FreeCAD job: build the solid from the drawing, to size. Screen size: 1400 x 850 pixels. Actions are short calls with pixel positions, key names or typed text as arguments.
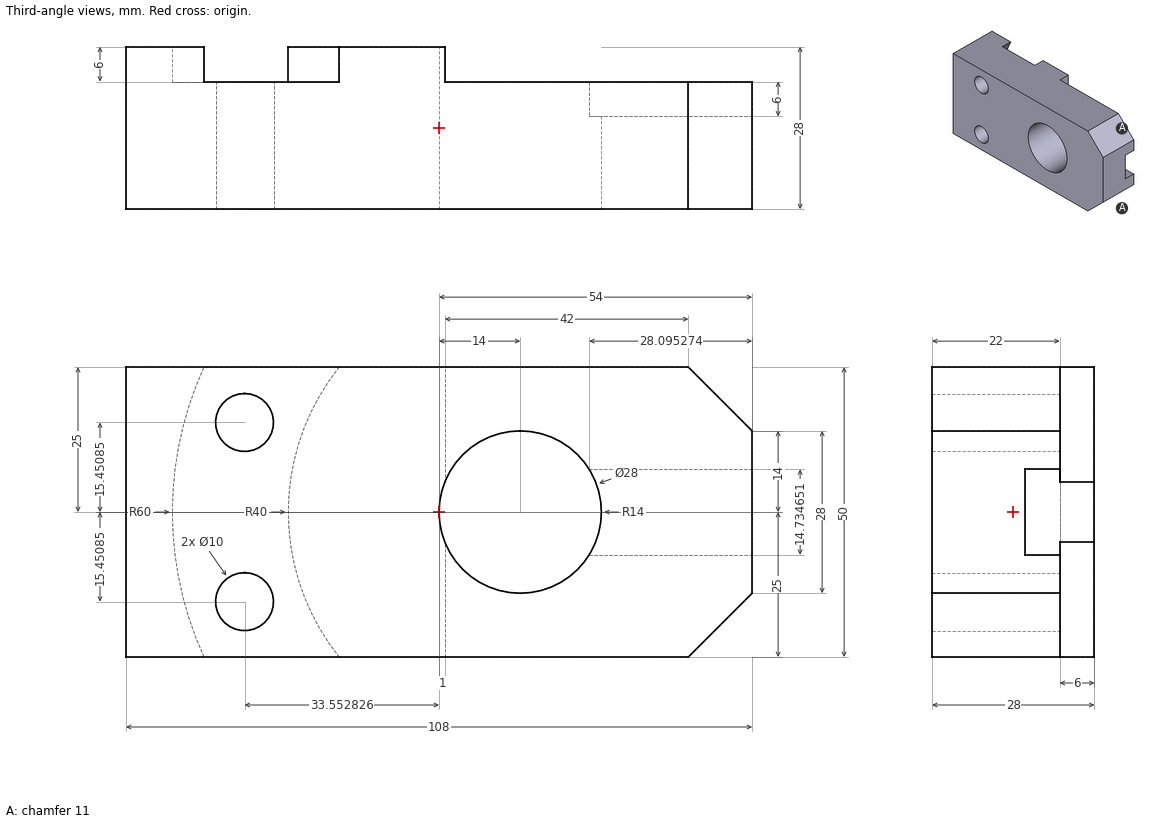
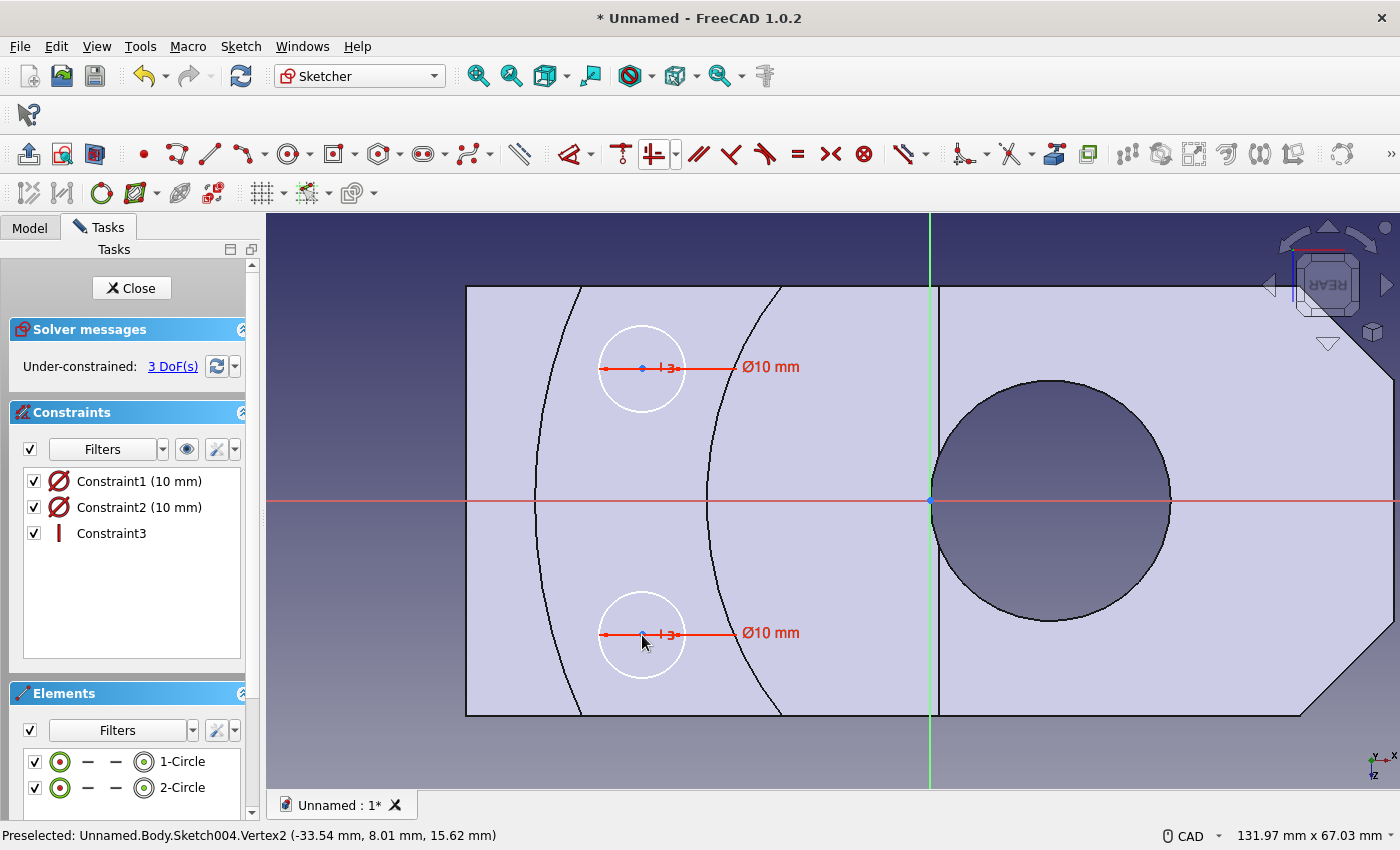
click(568, 154)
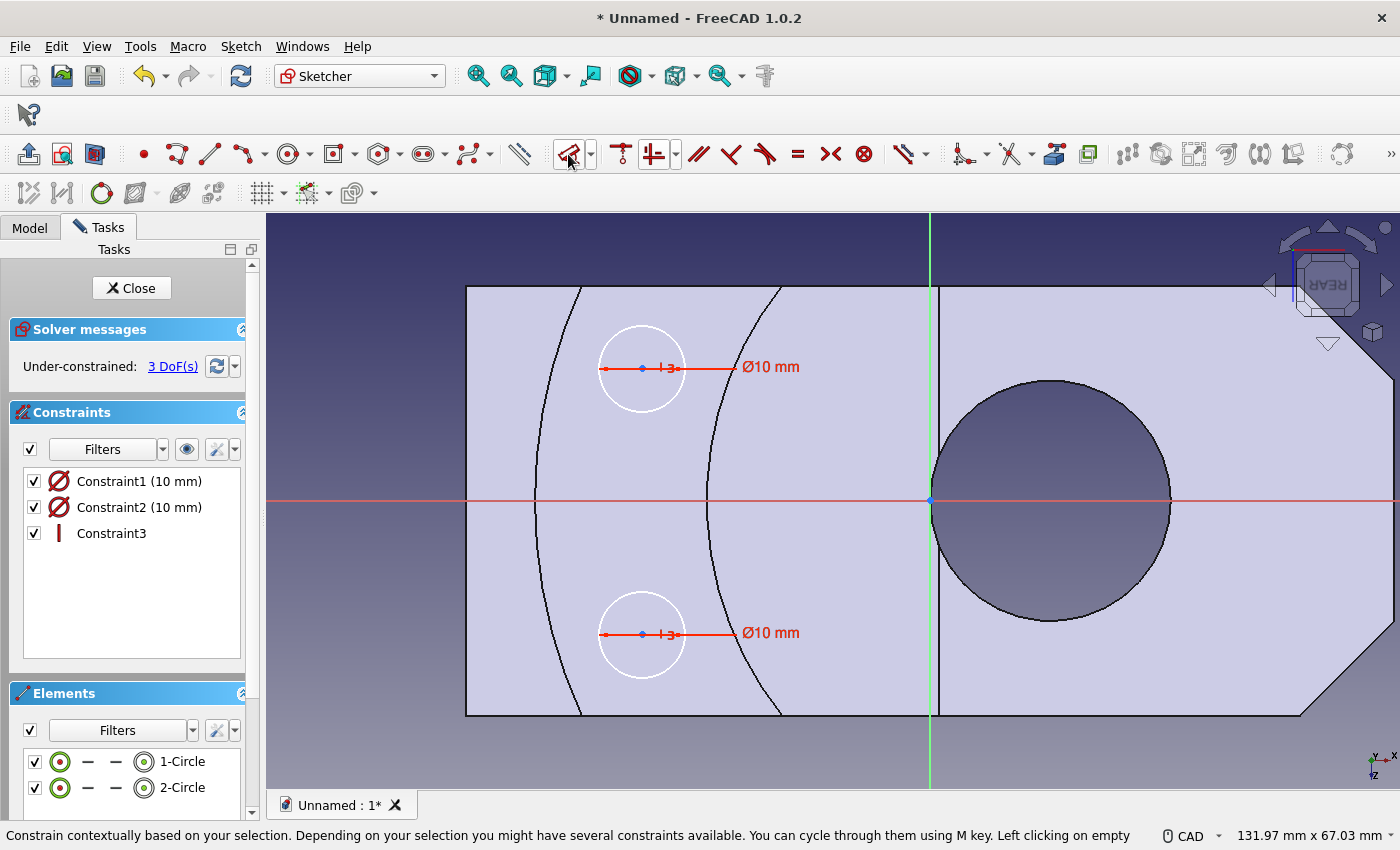
click(642, 369)
click(964, 435)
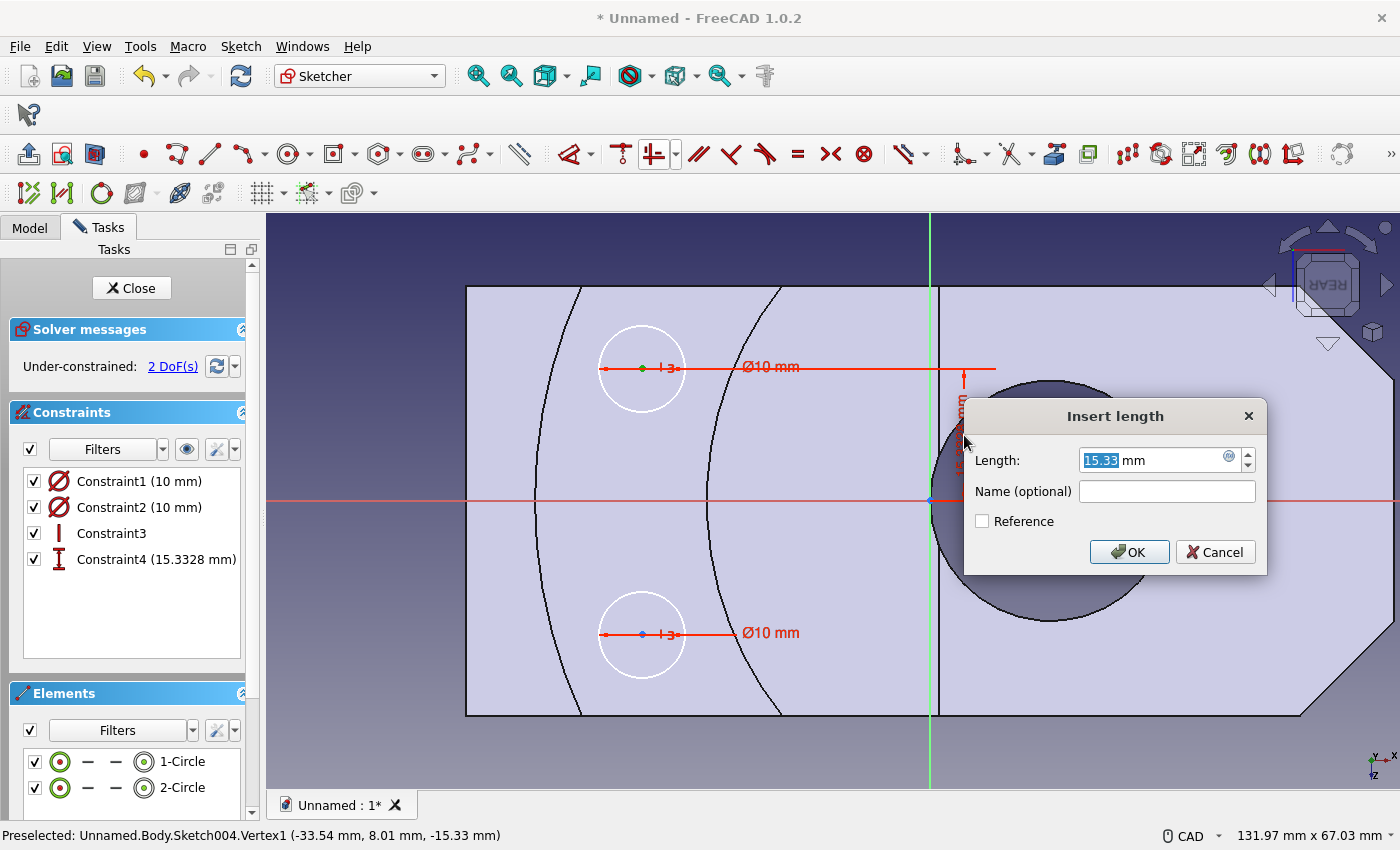
text(15.45085)
key(Return)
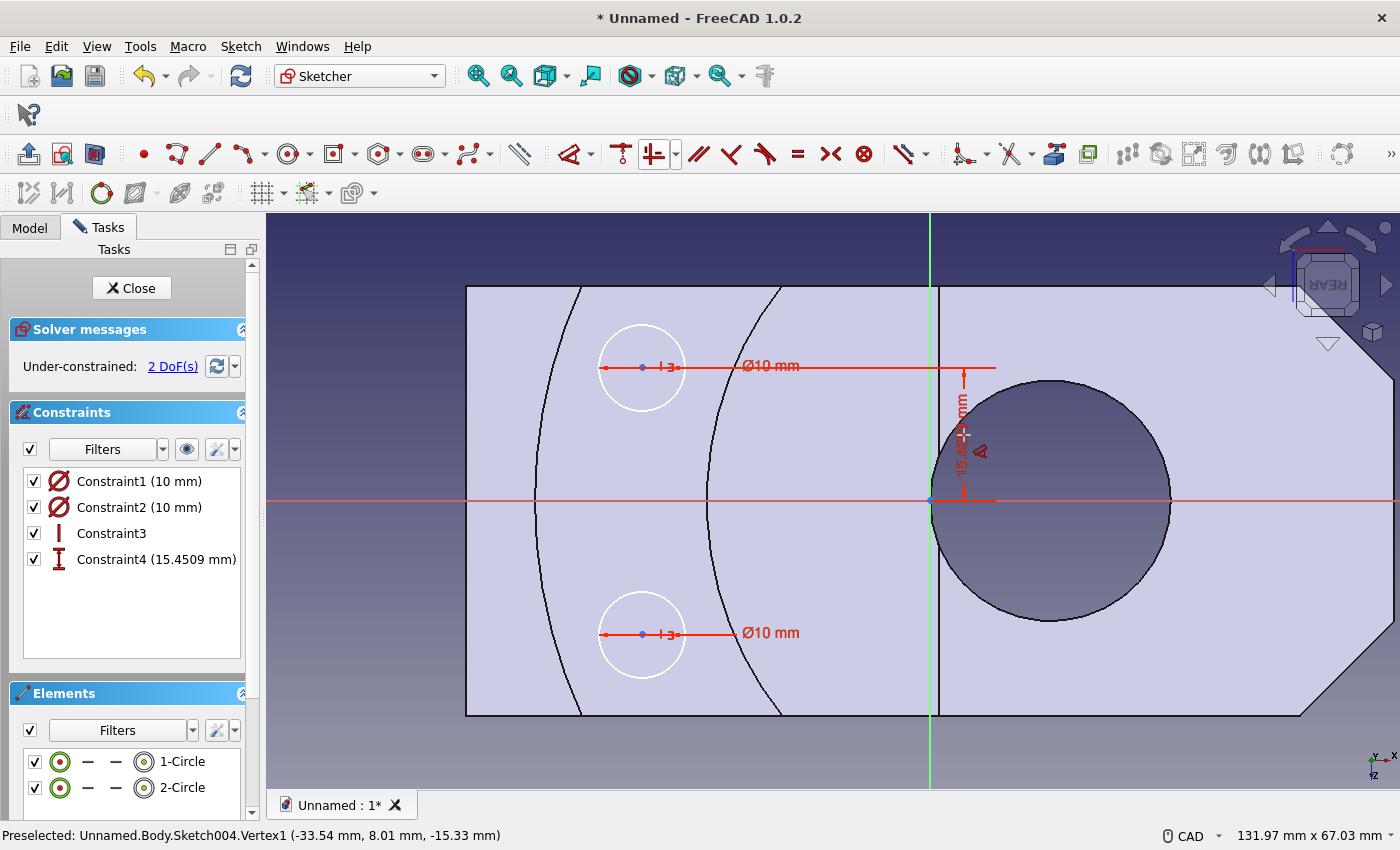
click(642, 635)
click(964, 568)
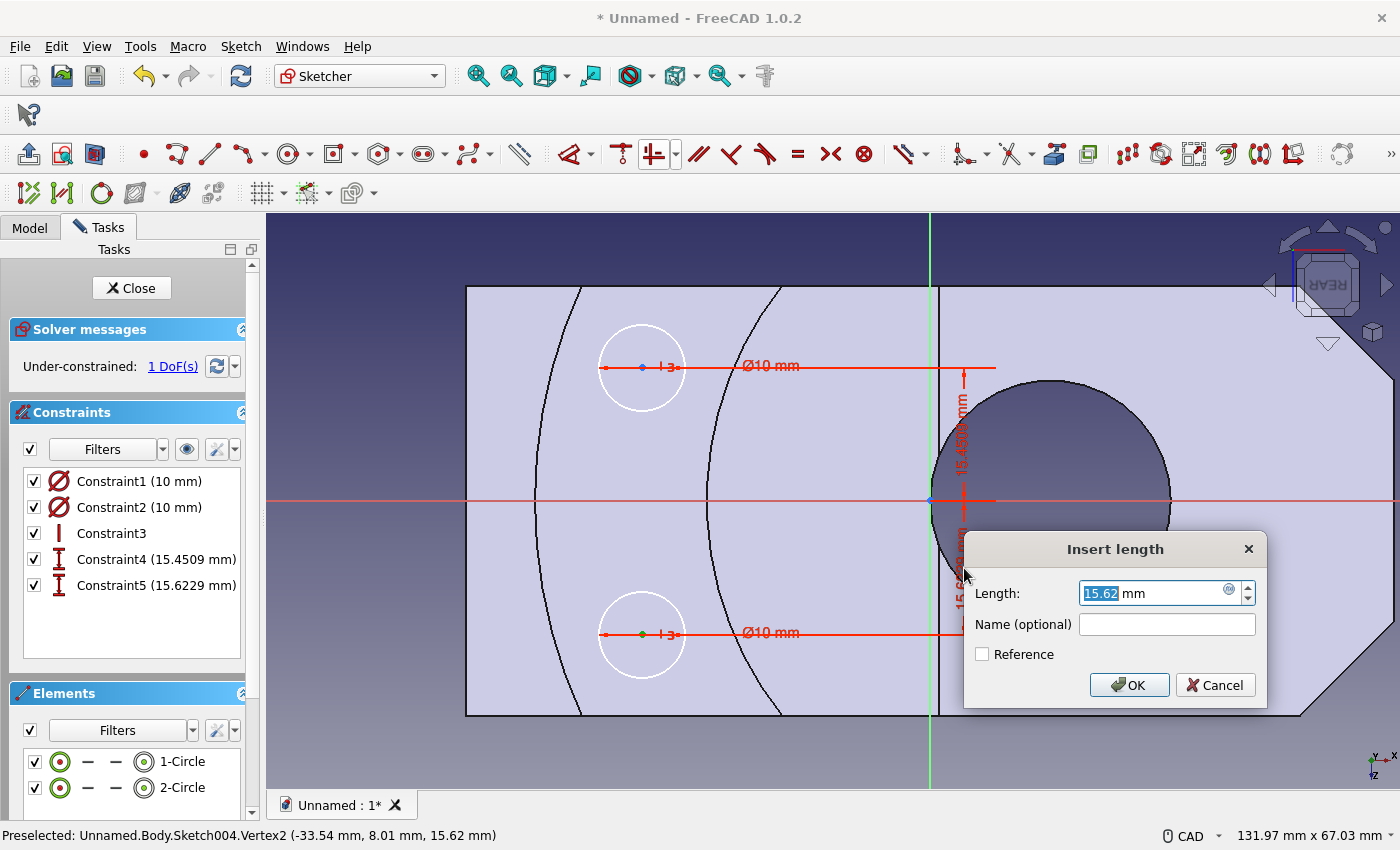
text(15.45085)
key(Return)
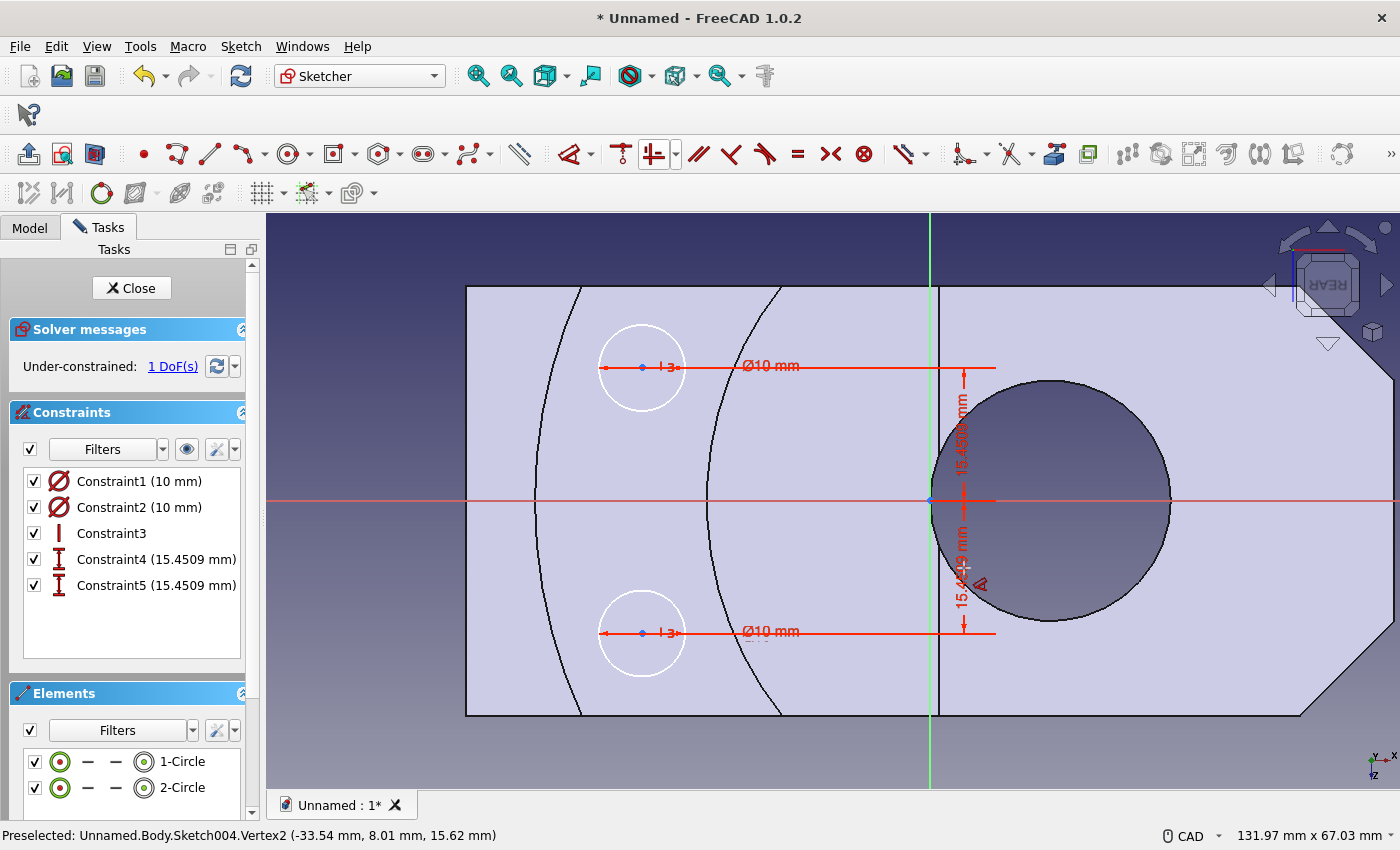
click(642, 368)
click(786, 334)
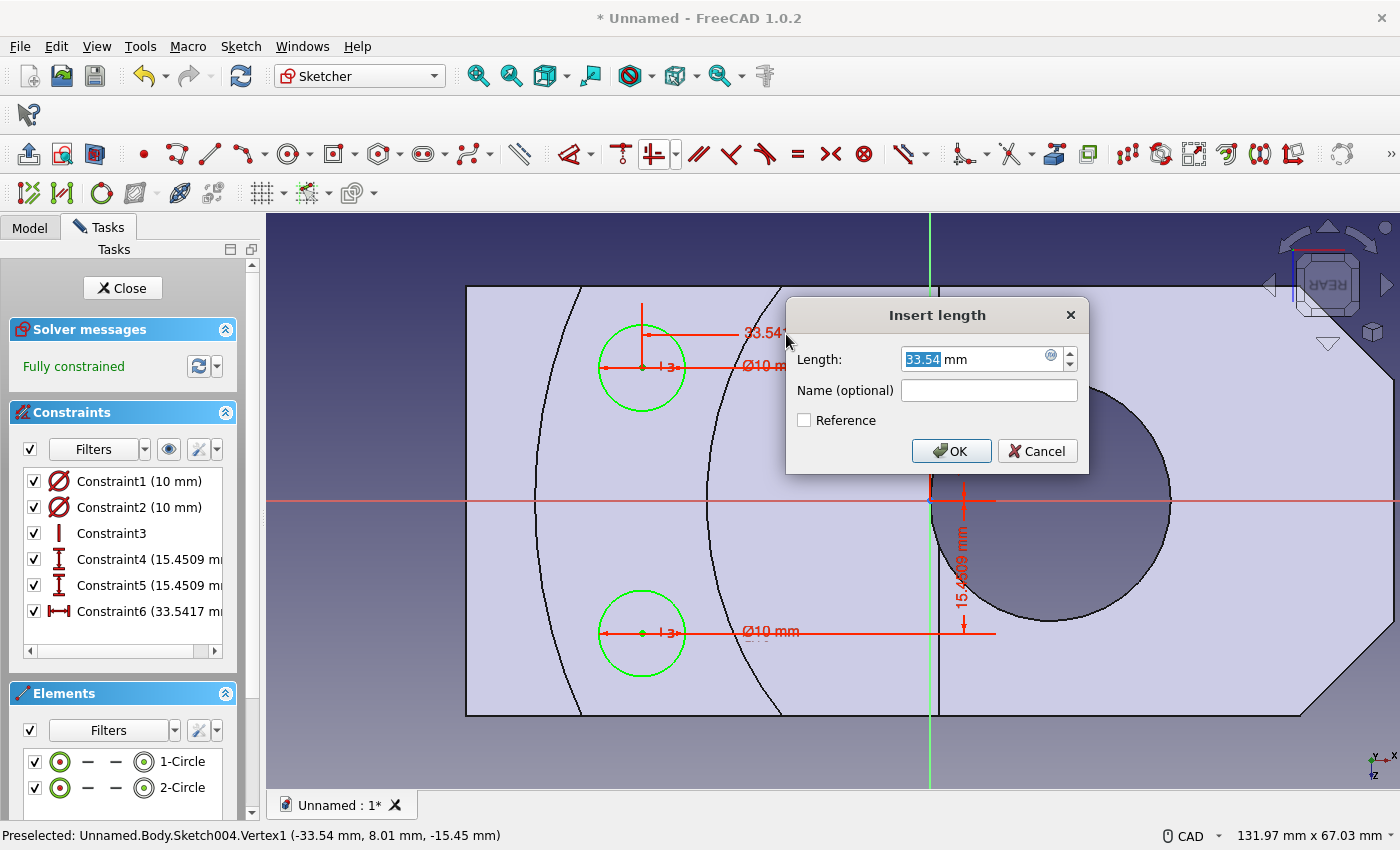
text(33.552826)
key(Return)
key(Escape)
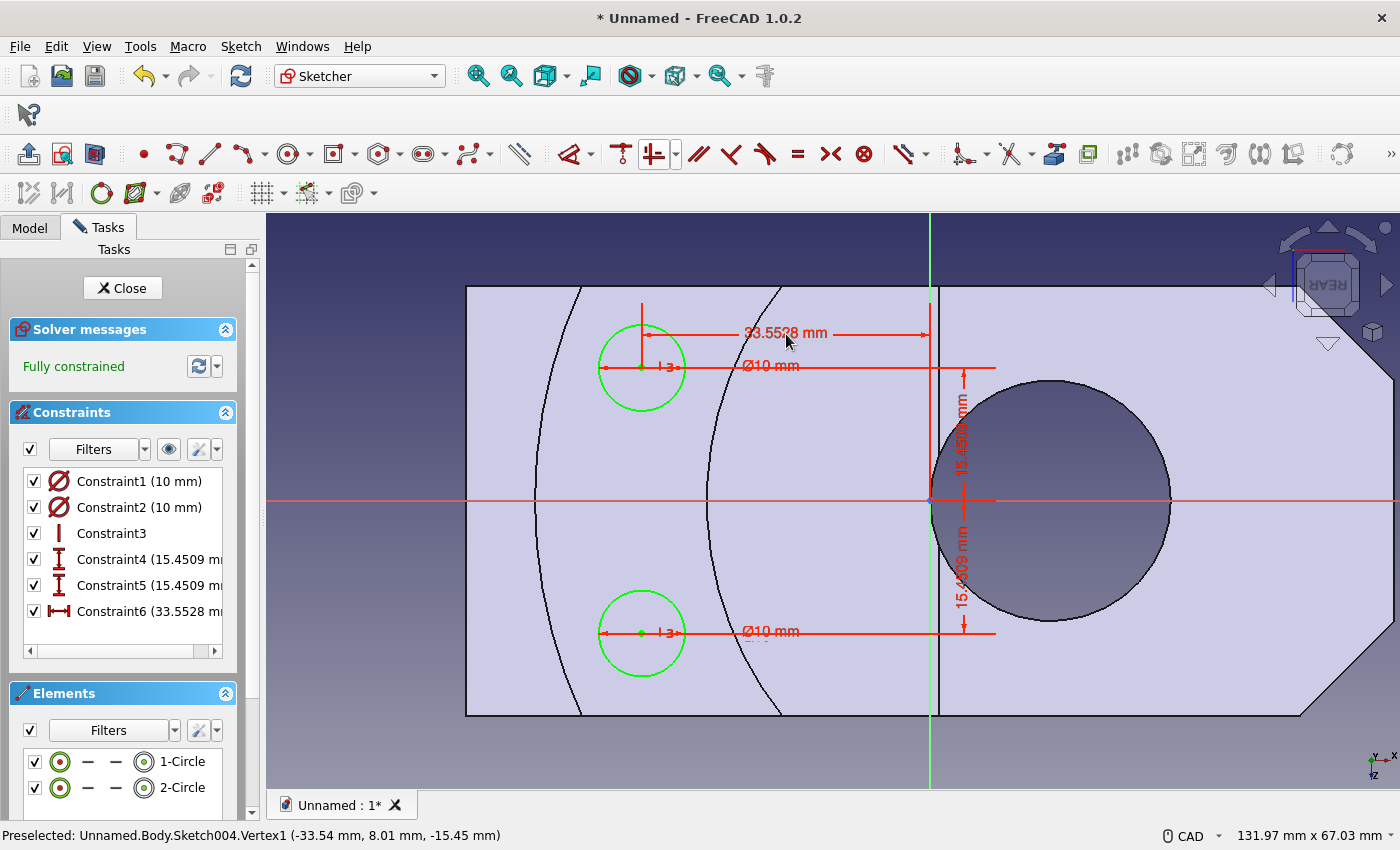
click(123, 288)